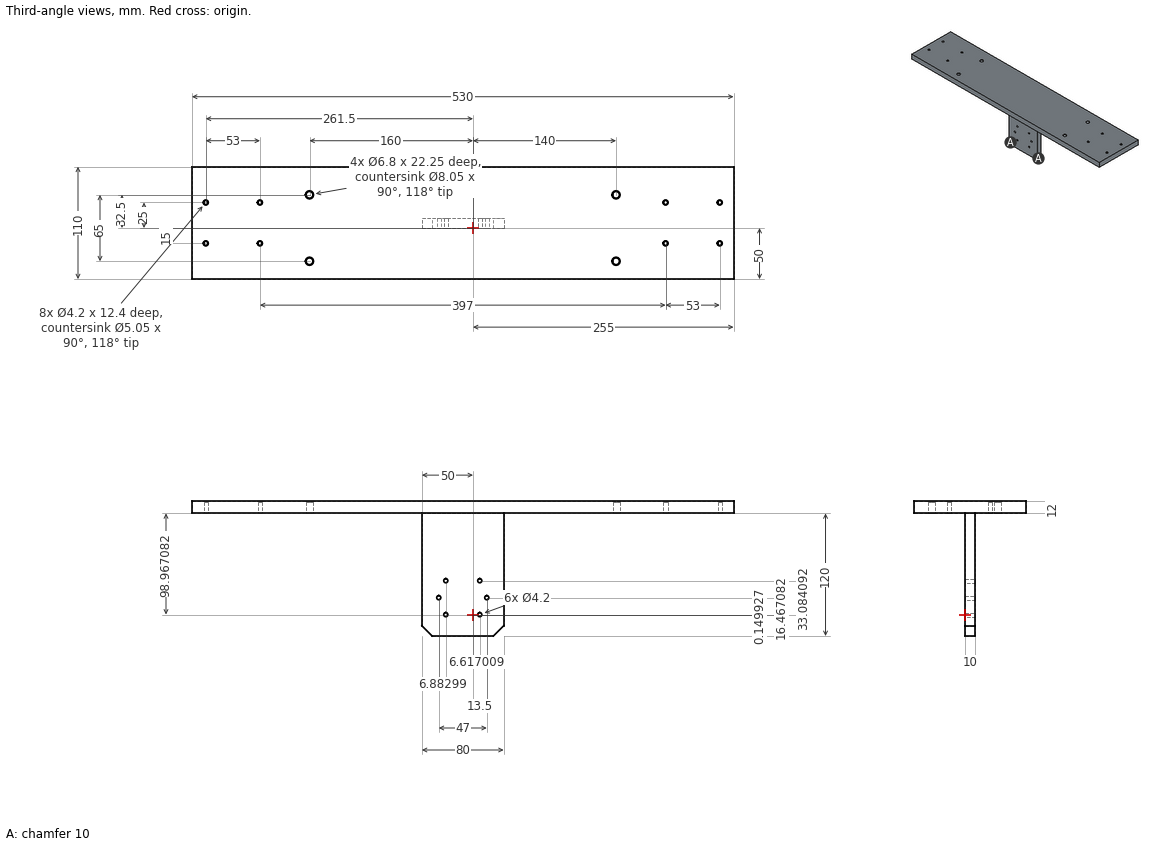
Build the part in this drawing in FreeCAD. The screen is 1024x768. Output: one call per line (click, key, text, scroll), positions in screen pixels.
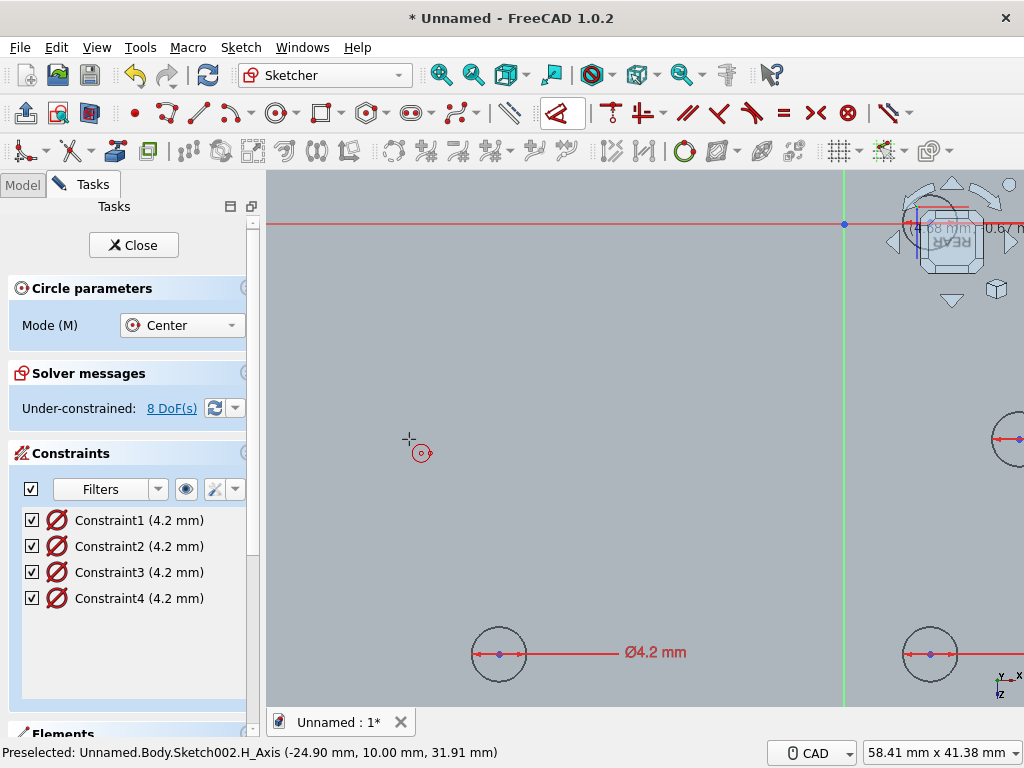
click(410, 438)
move(429, 419)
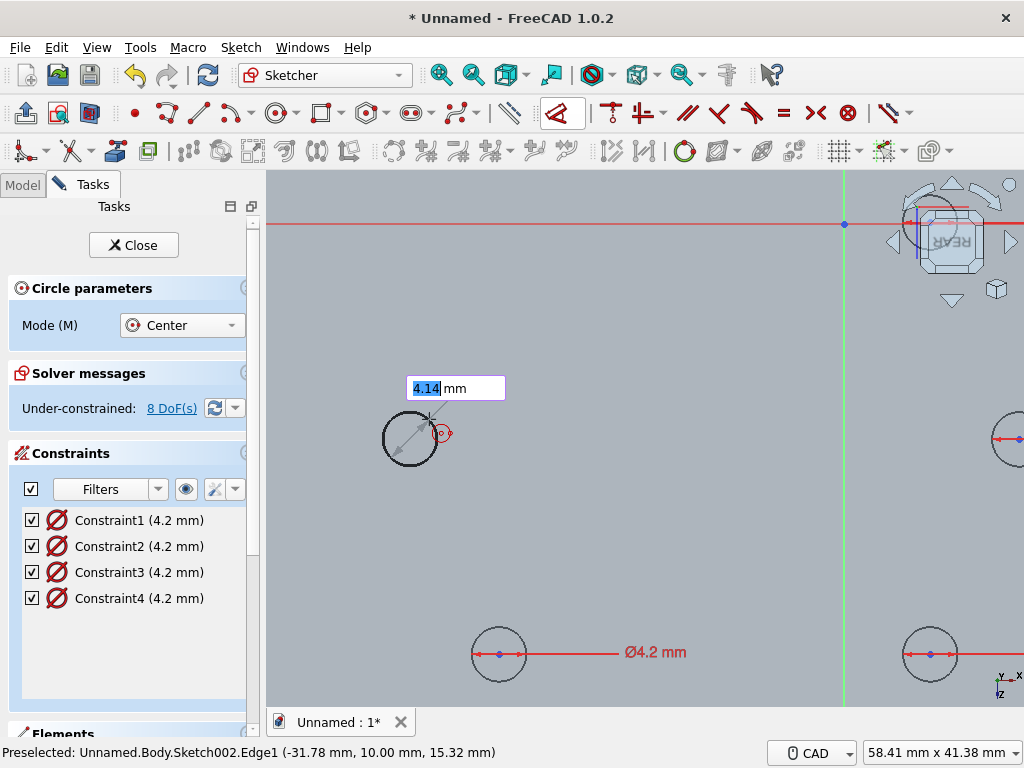
text(4.2)
key(Return)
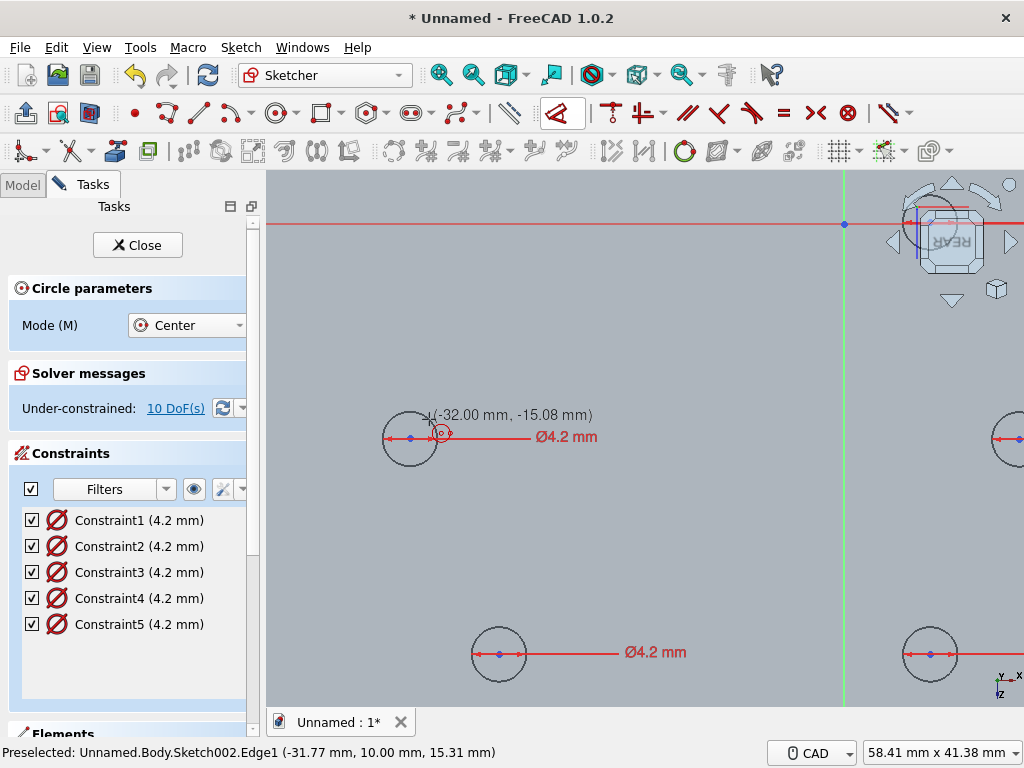
scroll(499, 222, up, 11)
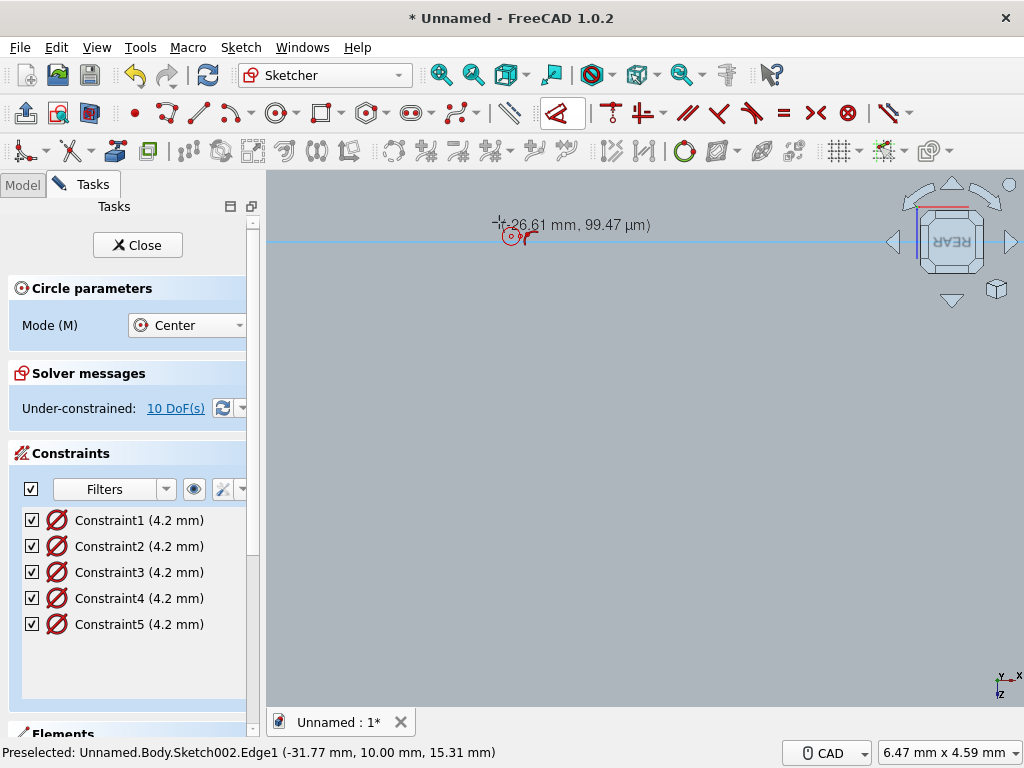
click(495, 224)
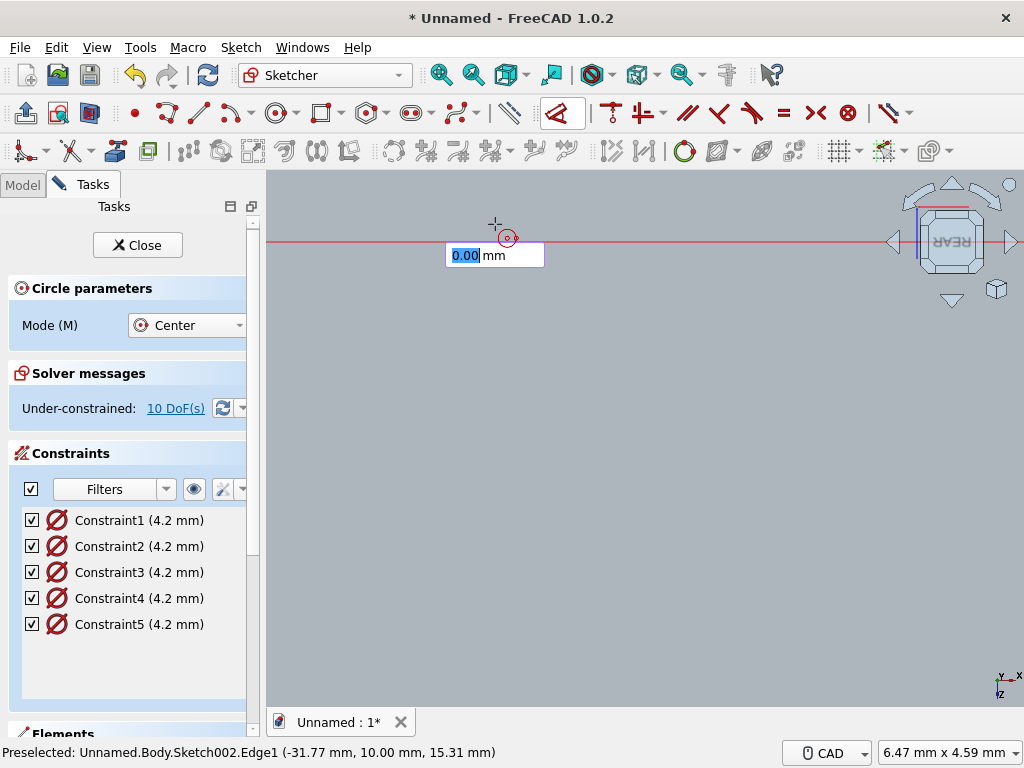
scroll(456, 326, down, 14)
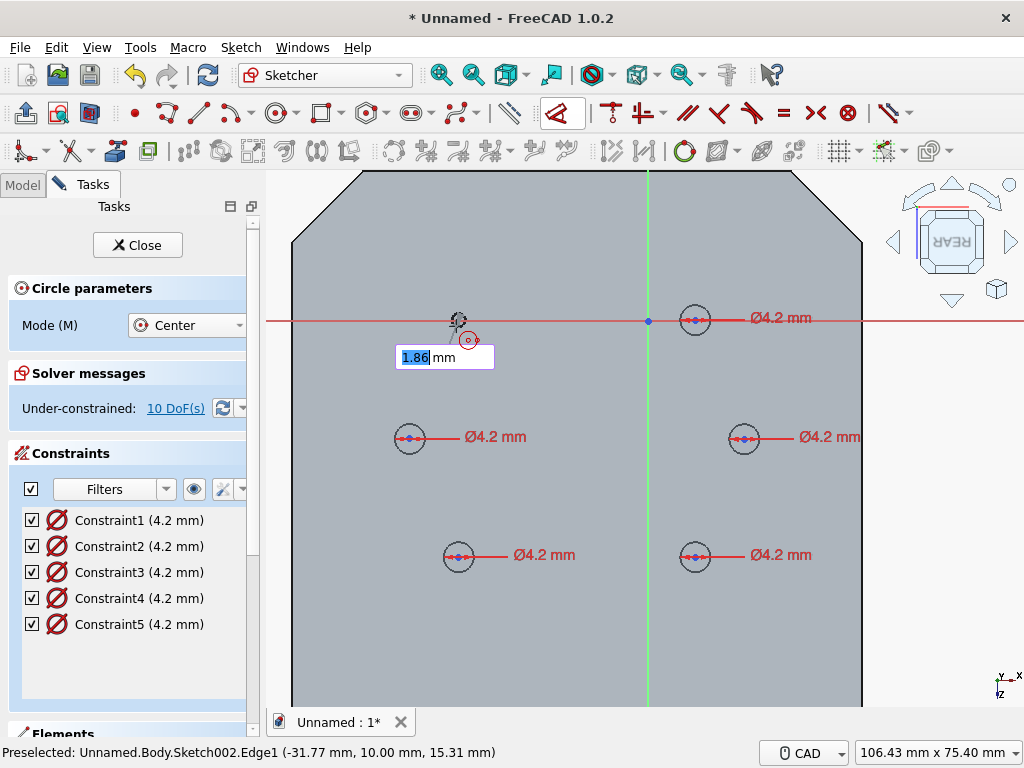
scroll(469, 310, up, 2)
move(469, 309)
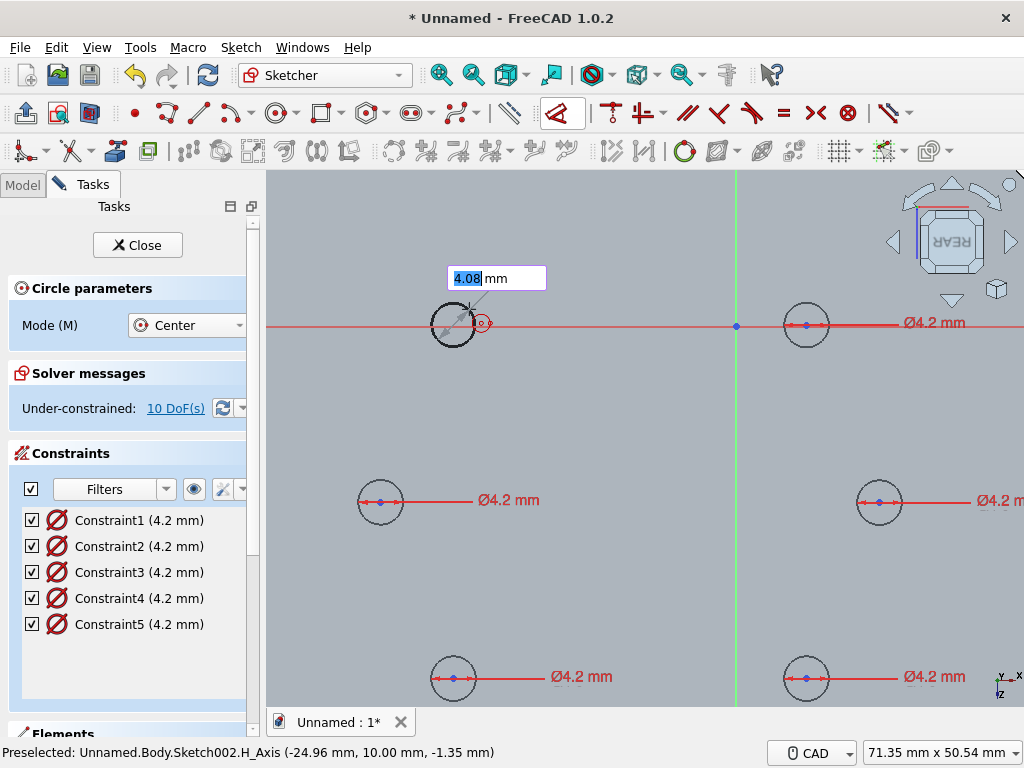
text(4.2)
key(Return)
key(Escape)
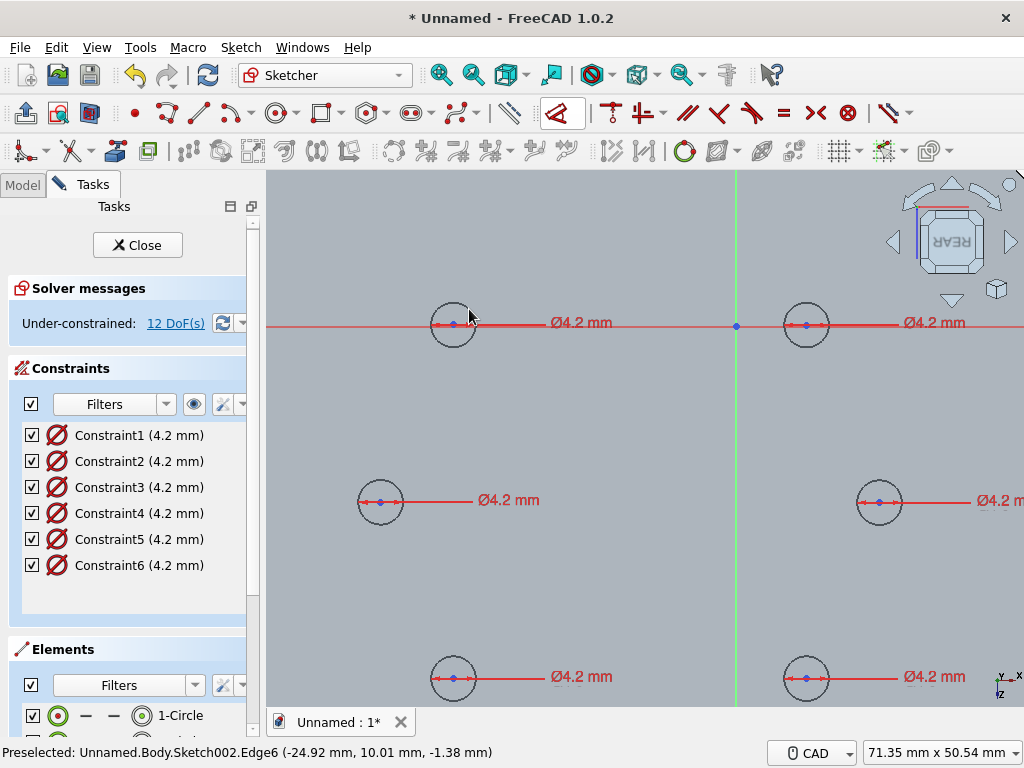
click(807, 325)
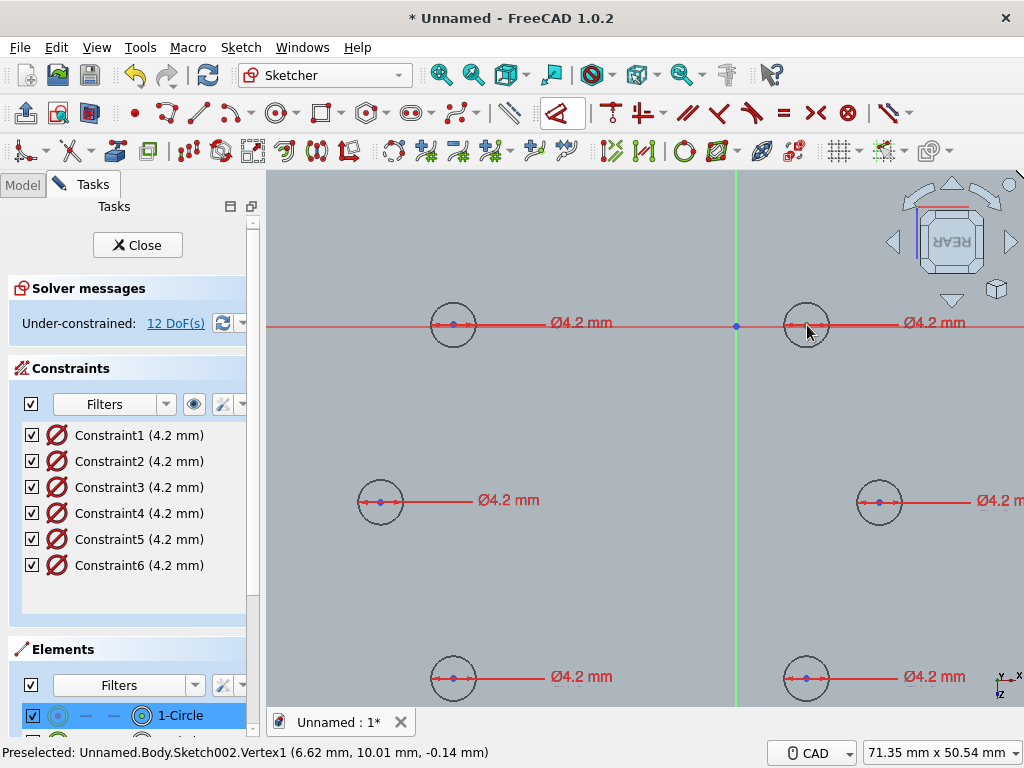
click(807, 679)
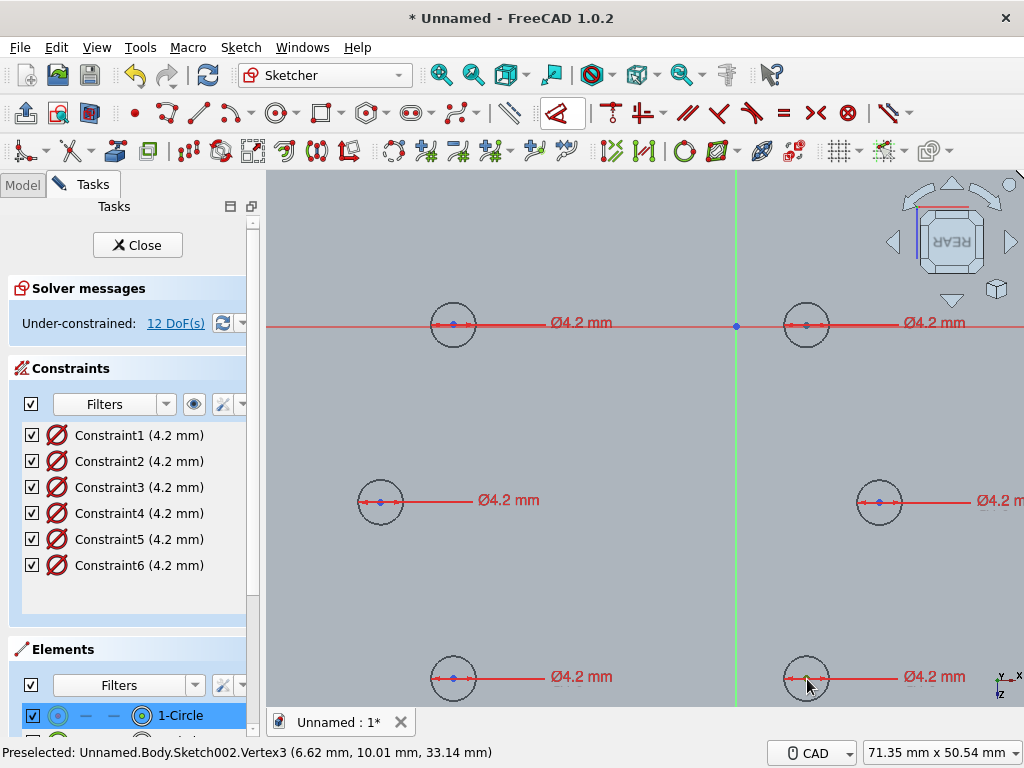
key(v)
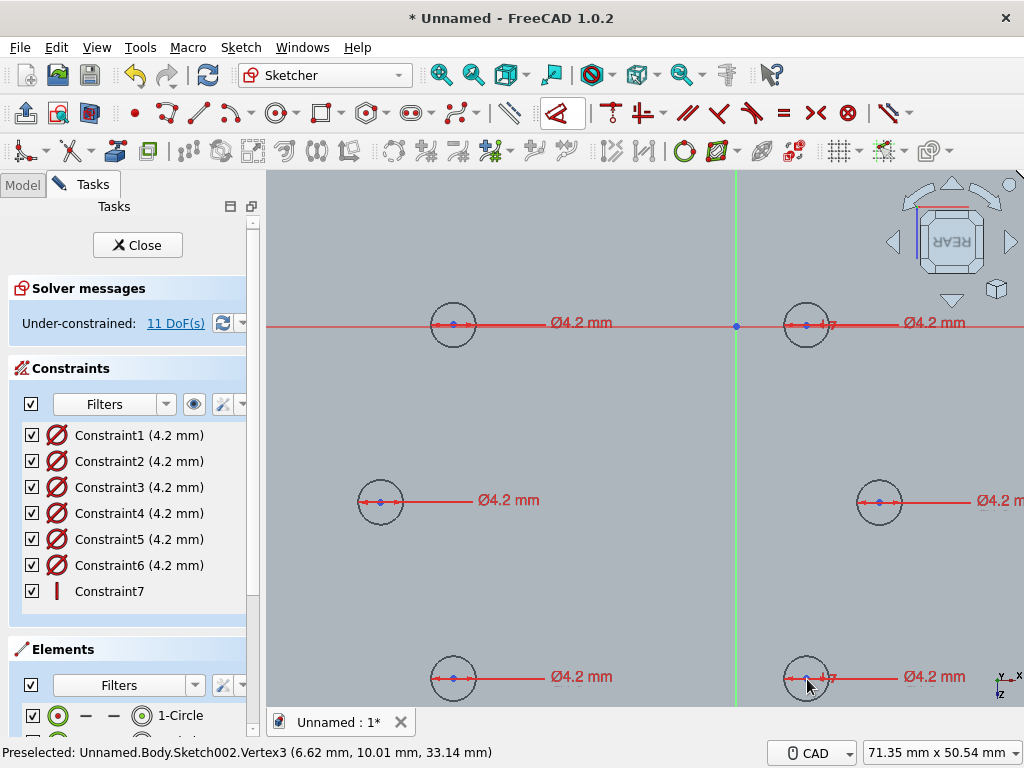
click(807, 679)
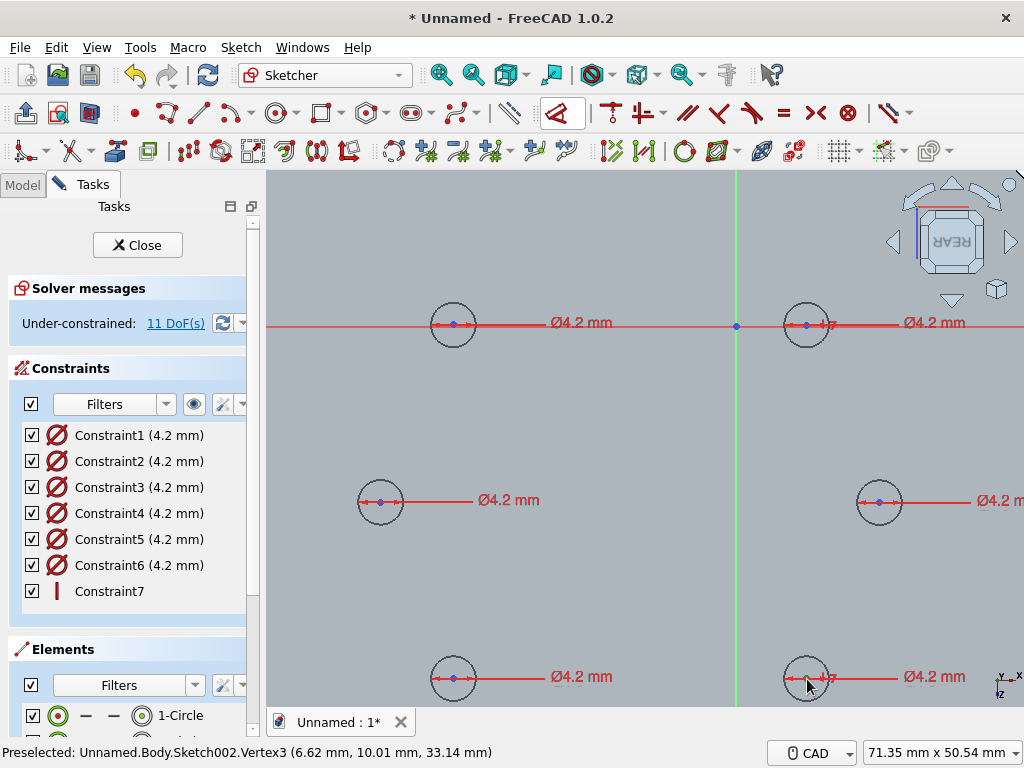
click(454, 679)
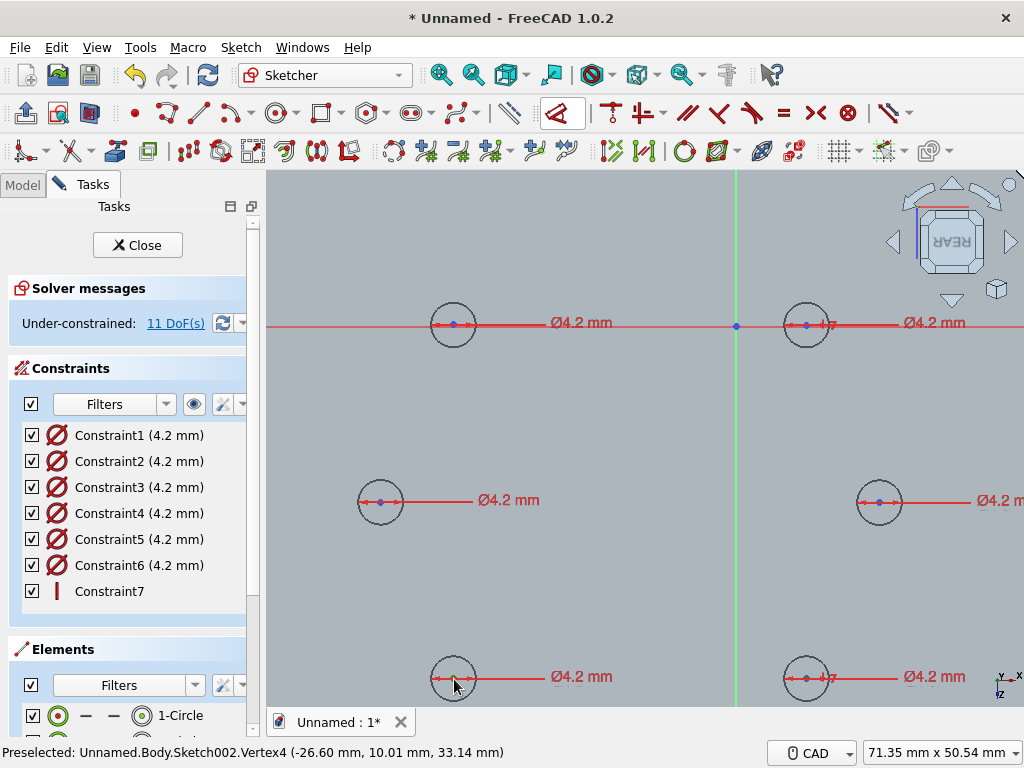
key(h)